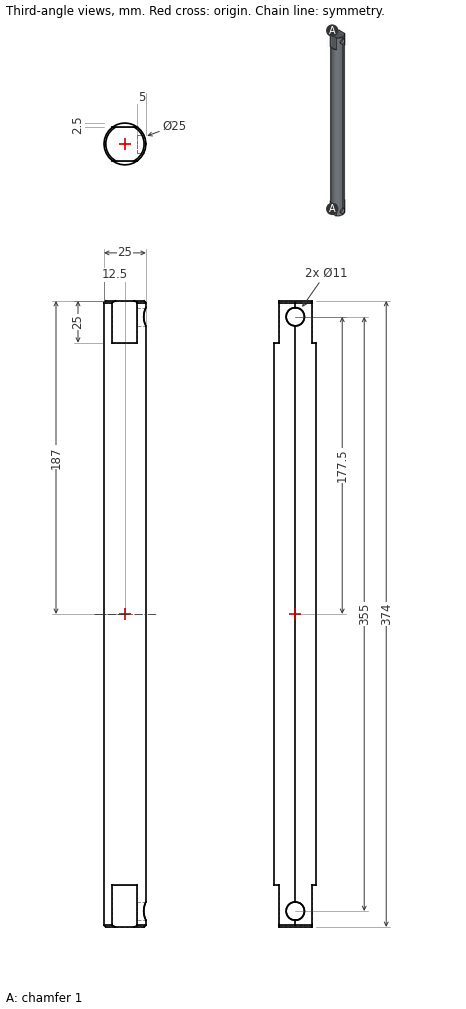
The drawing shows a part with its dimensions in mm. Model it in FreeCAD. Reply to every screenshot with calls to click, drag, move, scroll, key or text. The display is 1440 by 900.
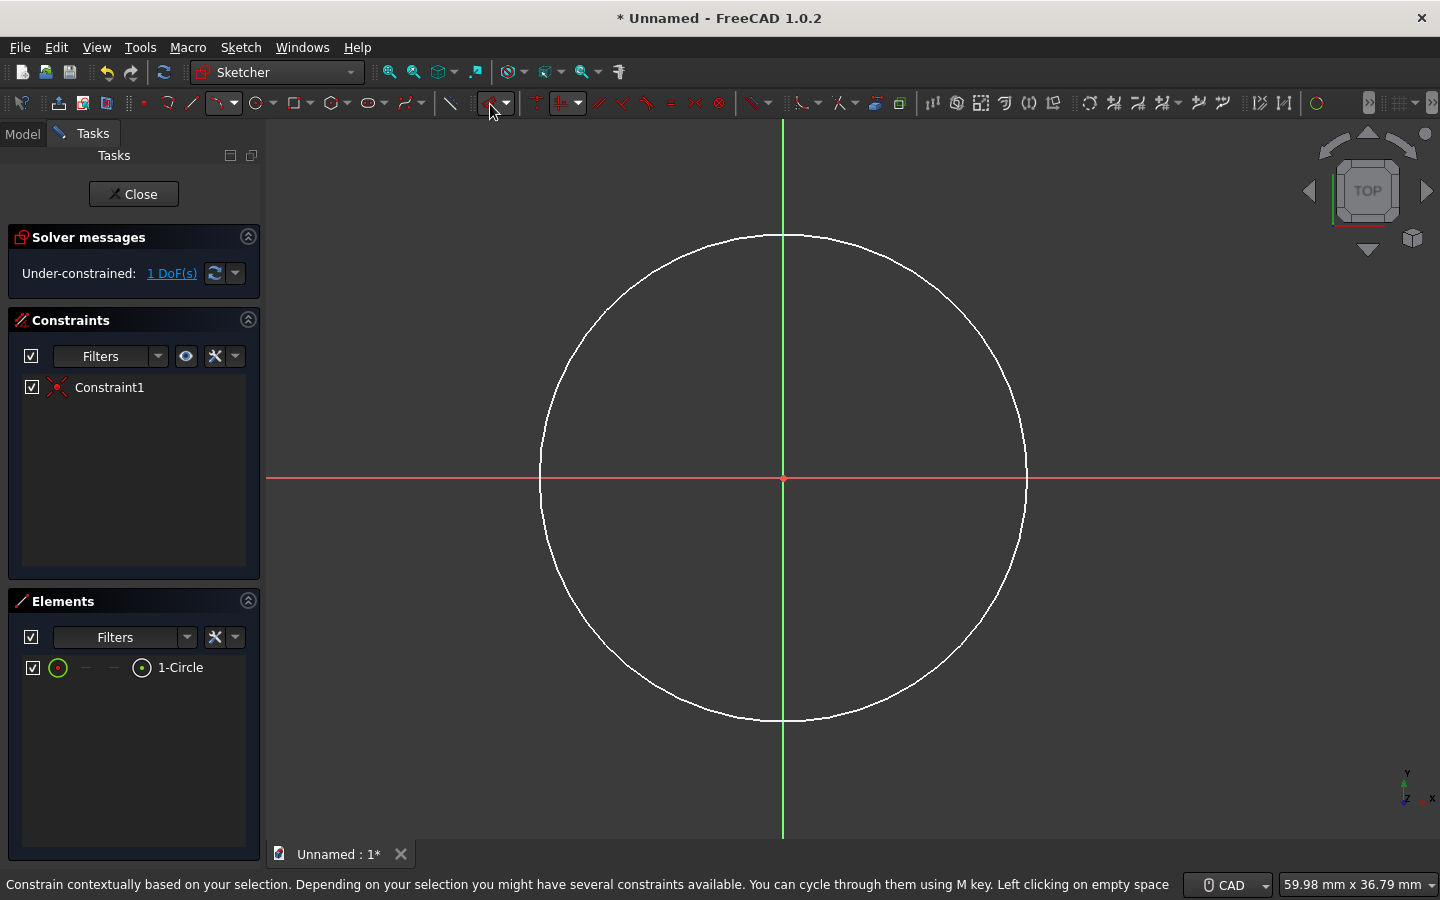
click(955, 305)
click(978, 282)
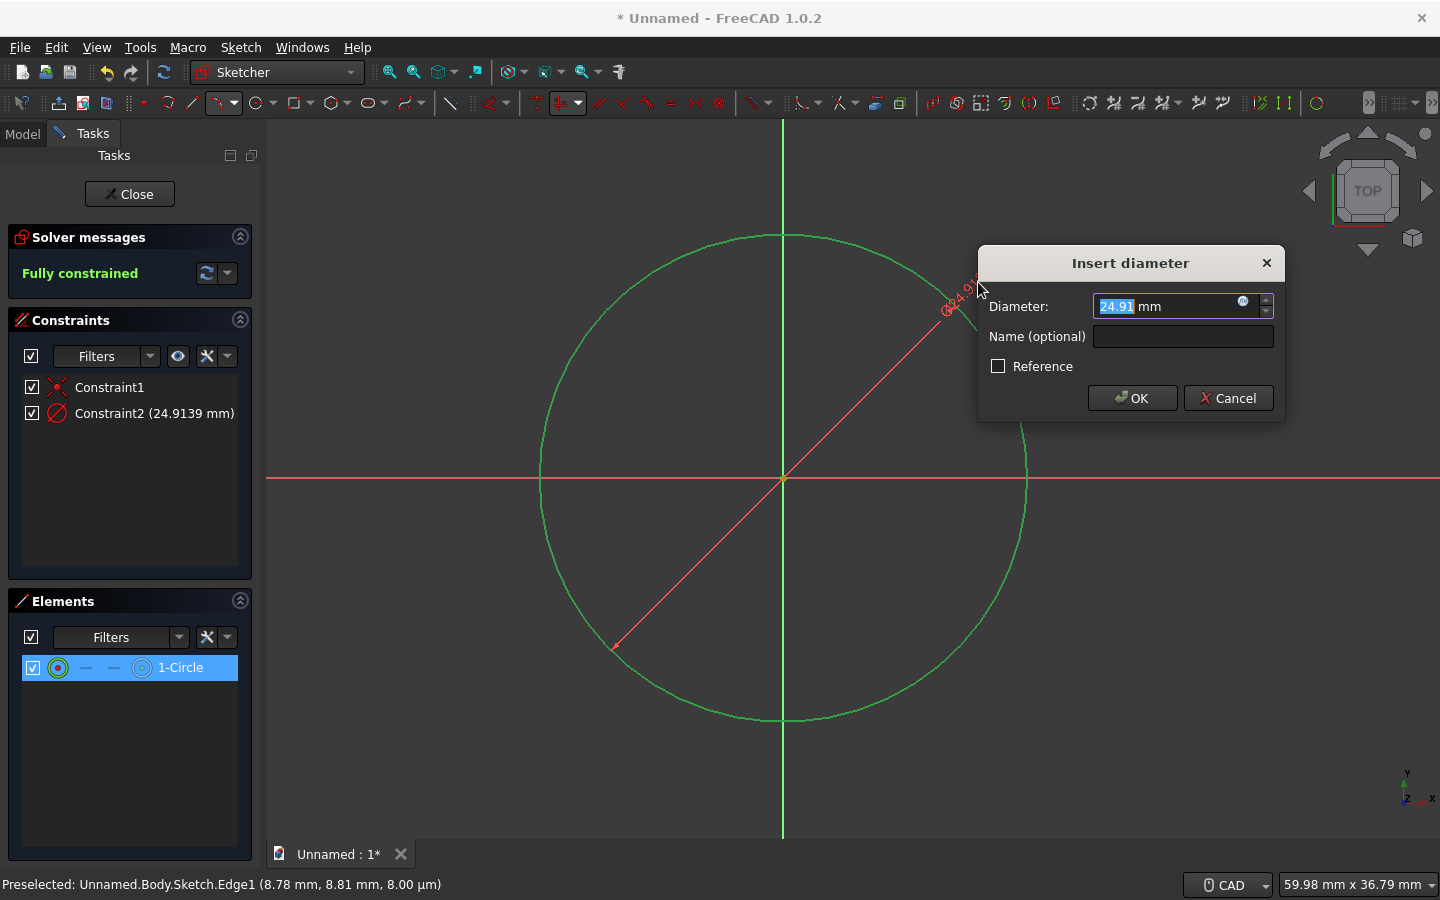
text(25)
key(Return)
key(Escape)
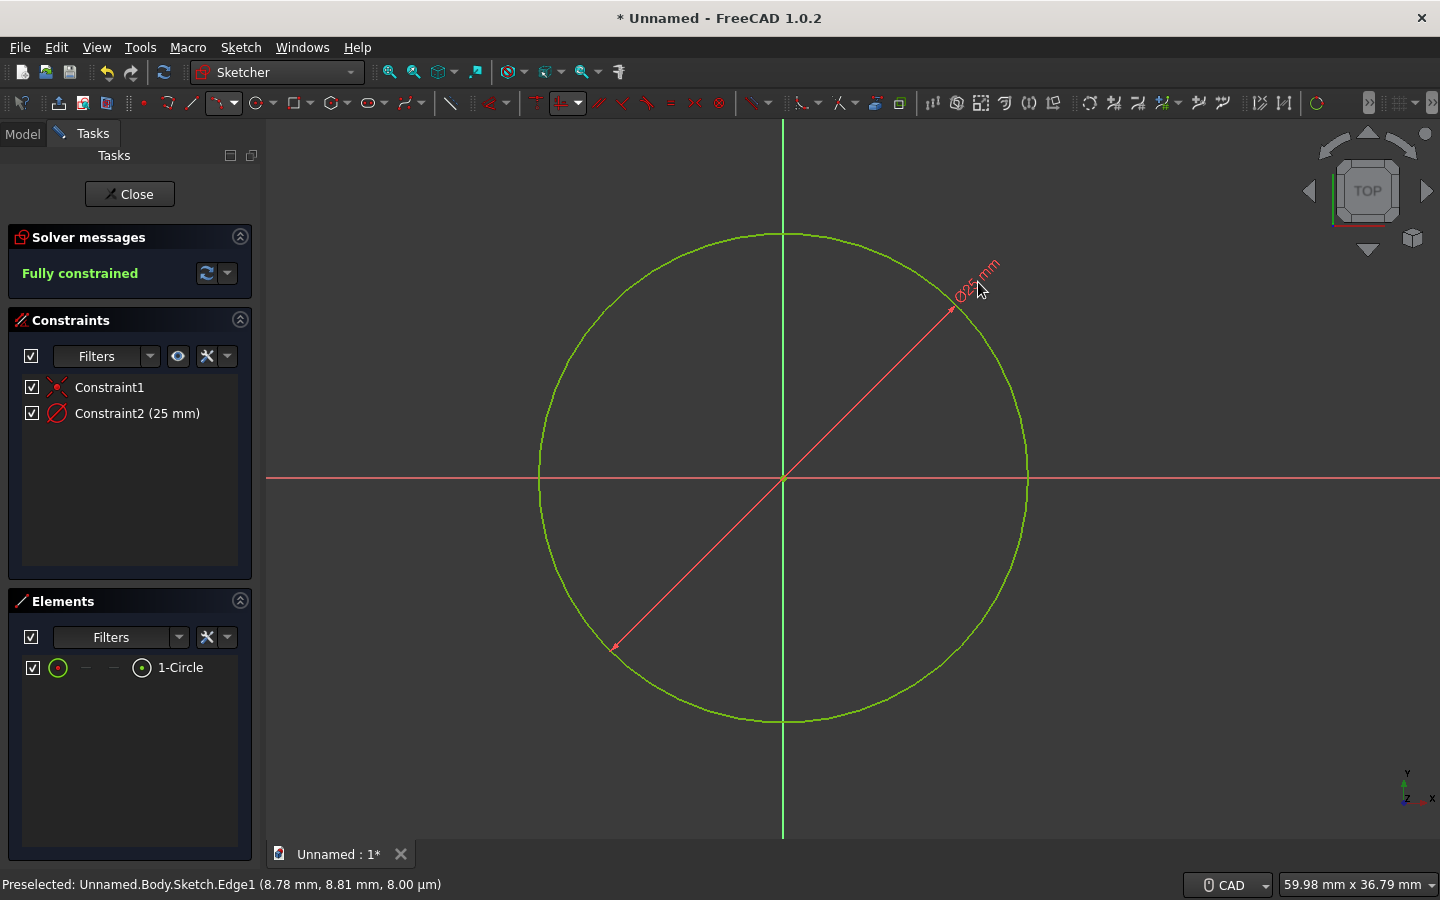
click(130, 194)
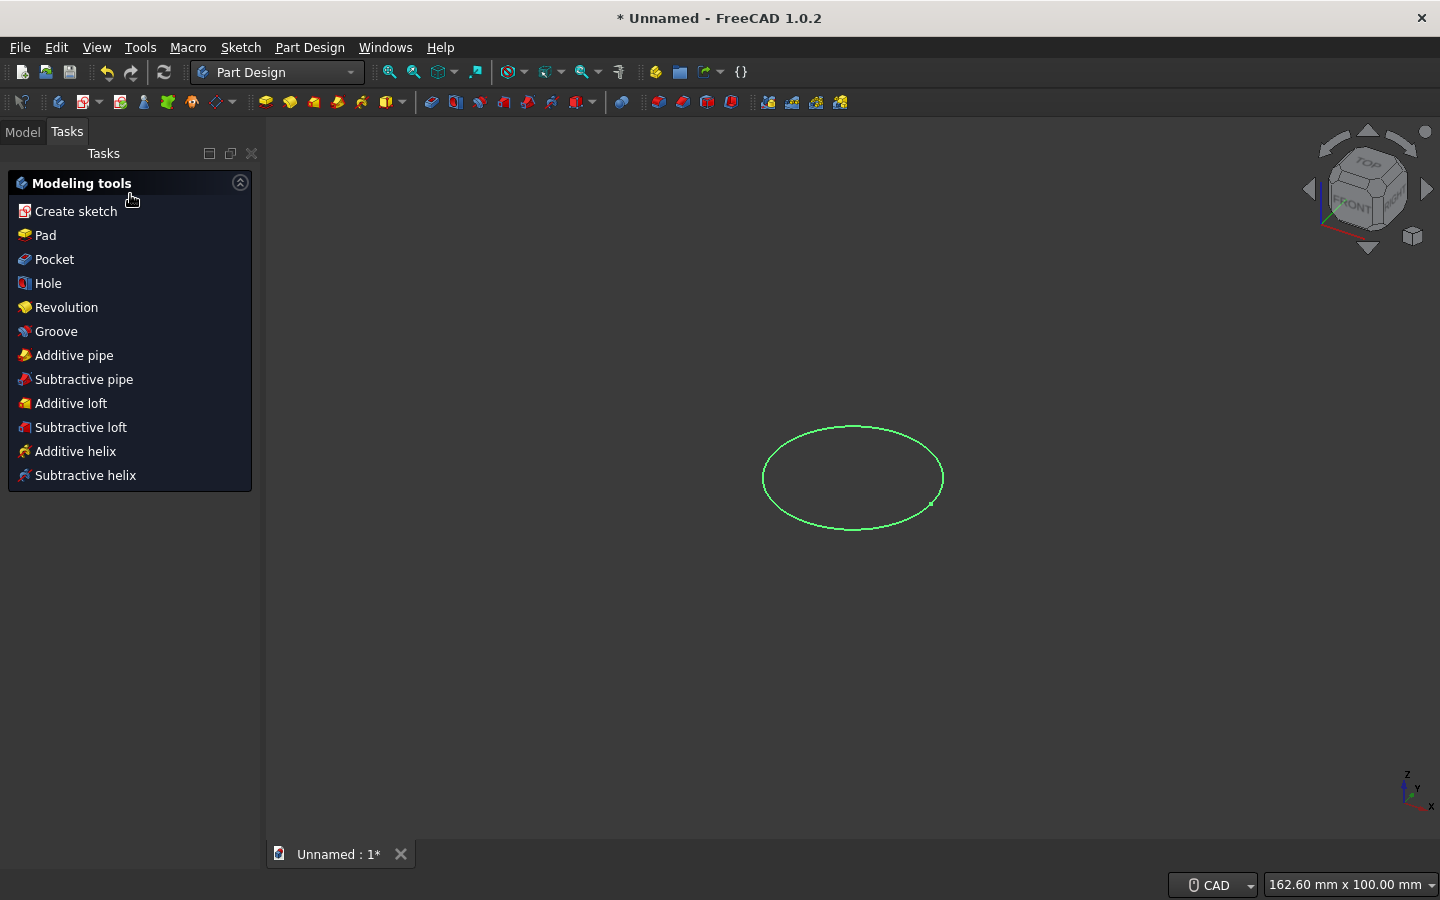
click(266, 102)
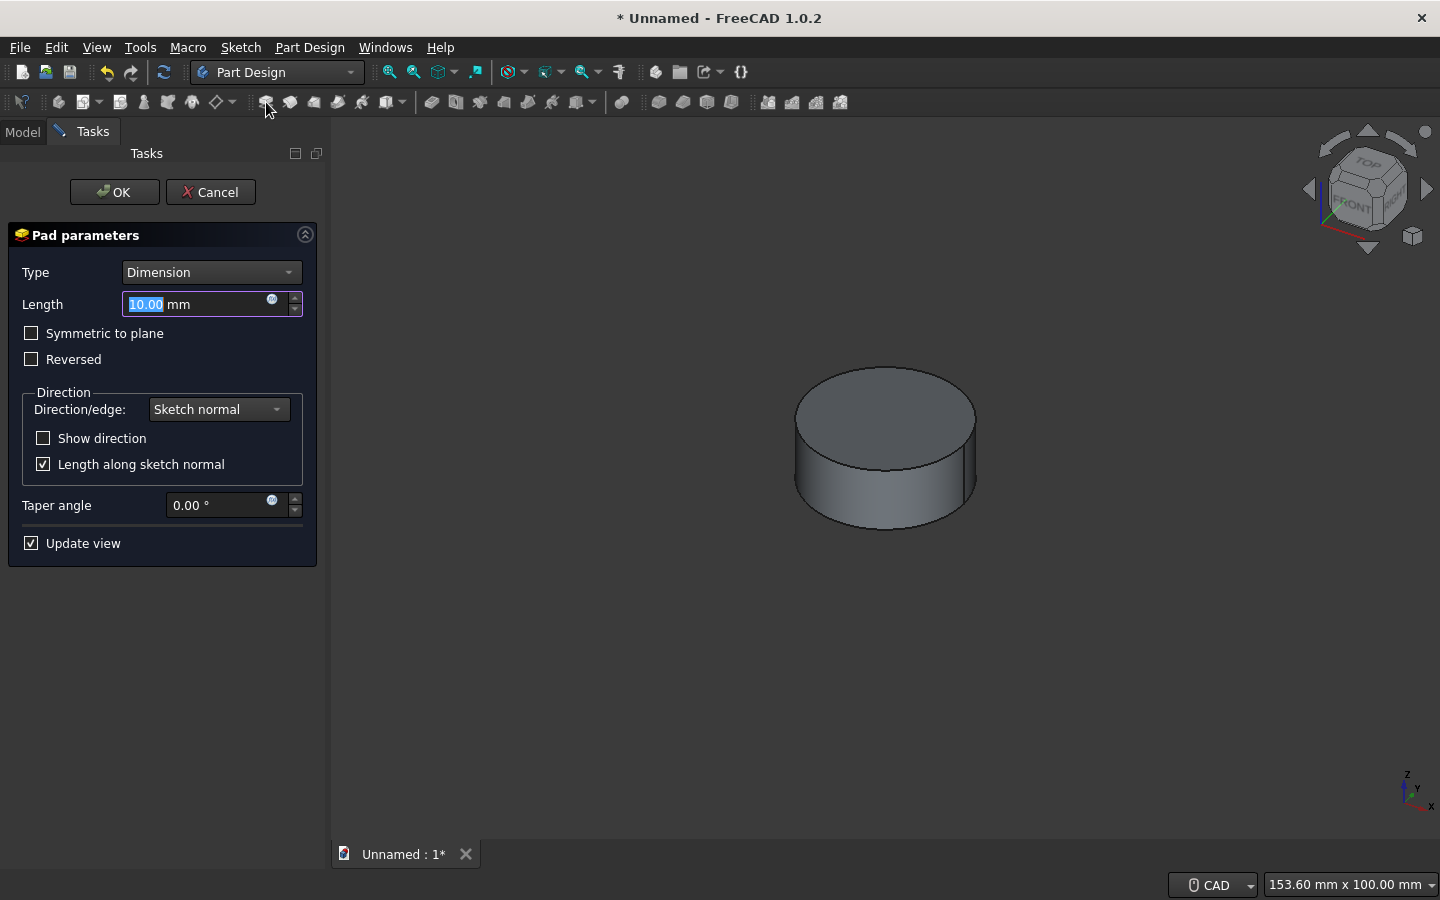
text(374)
key(Tab)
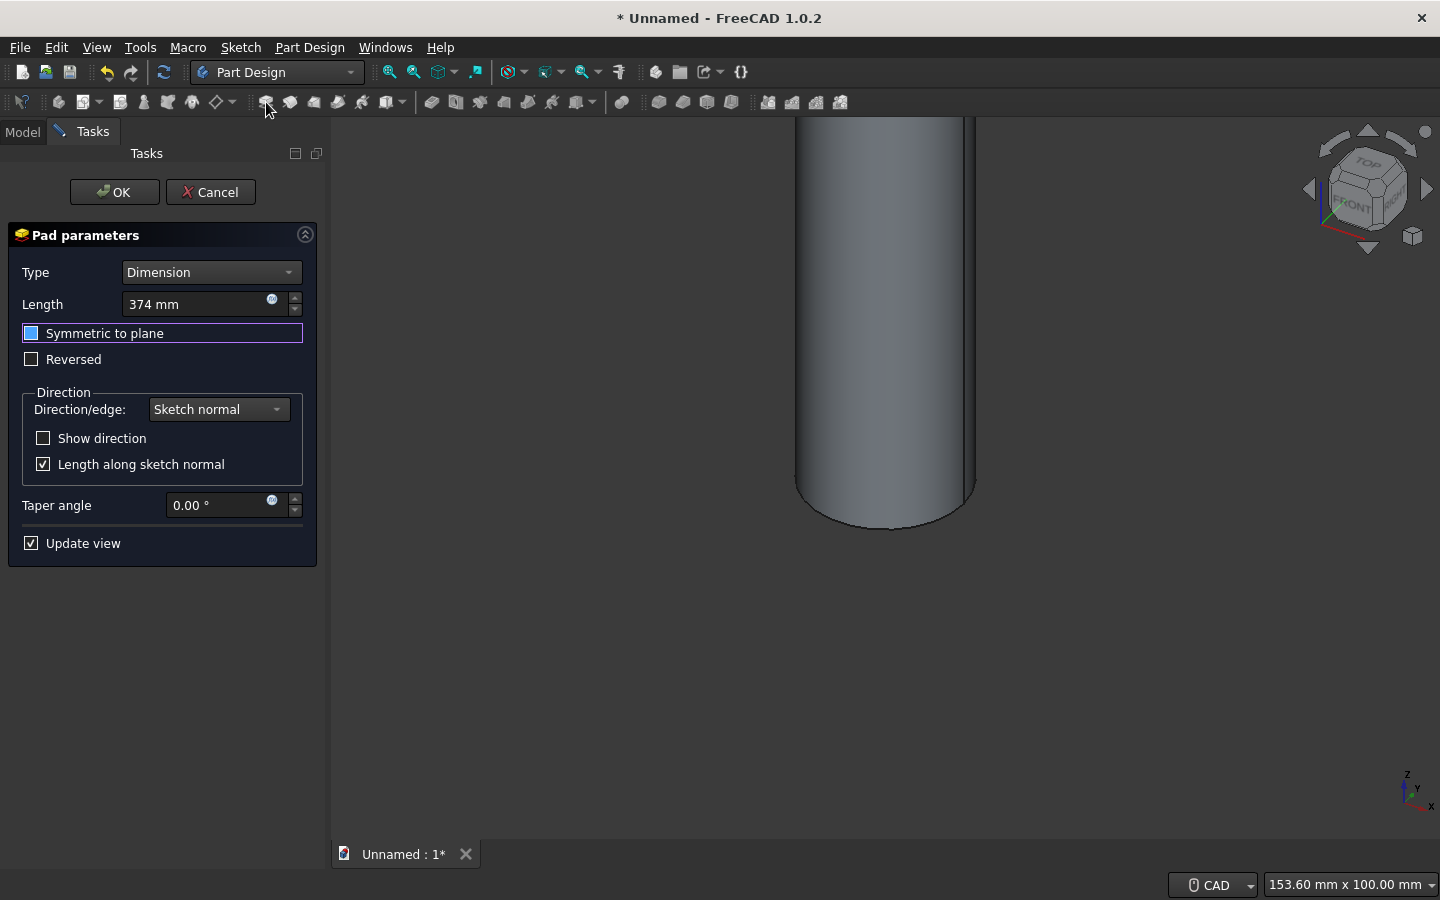
click(30, 333)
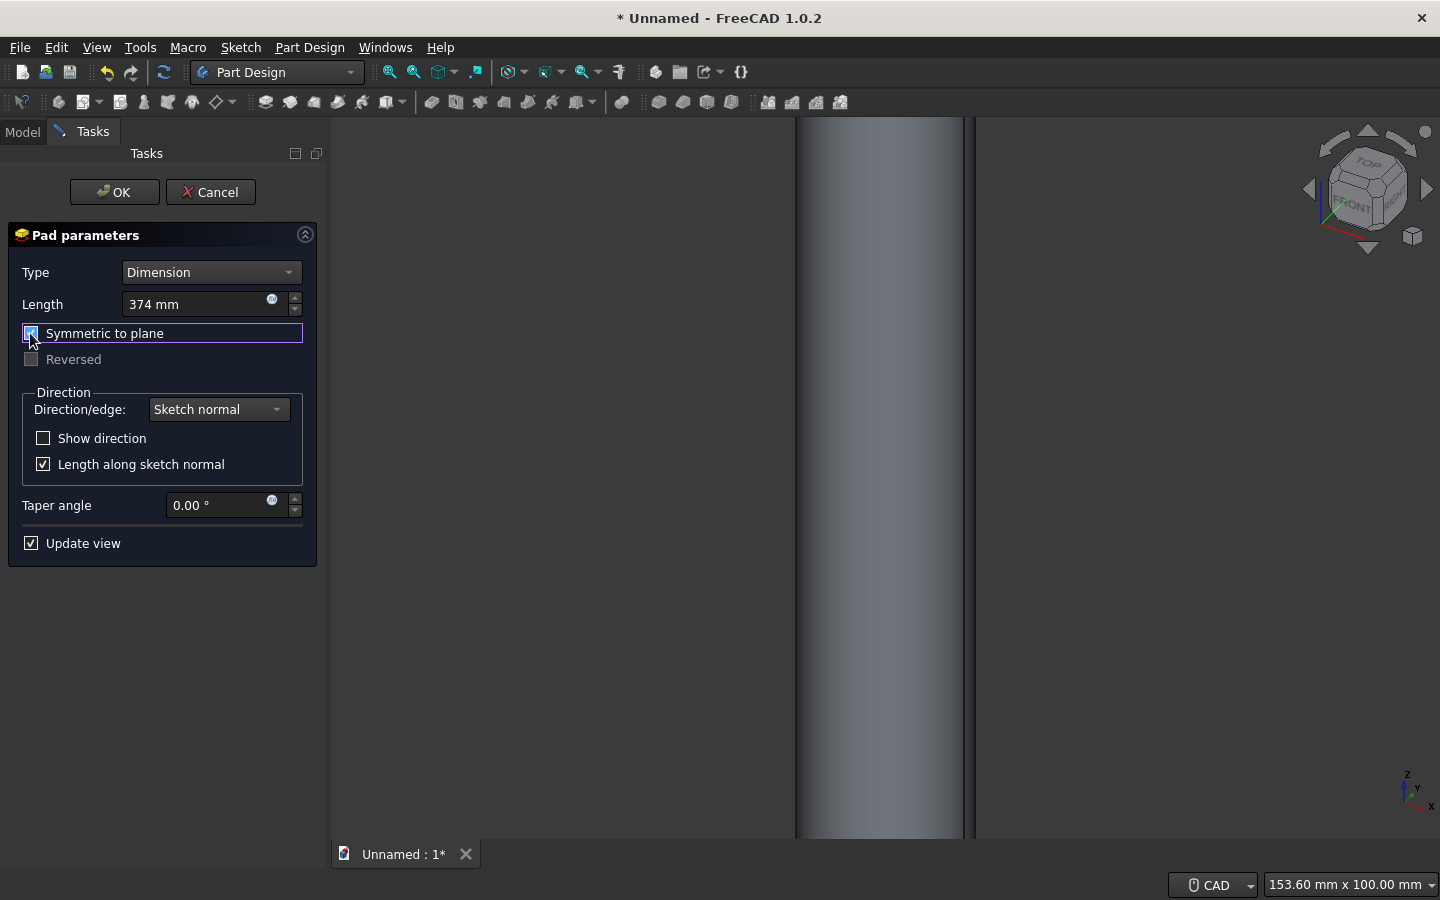
click(115, 192)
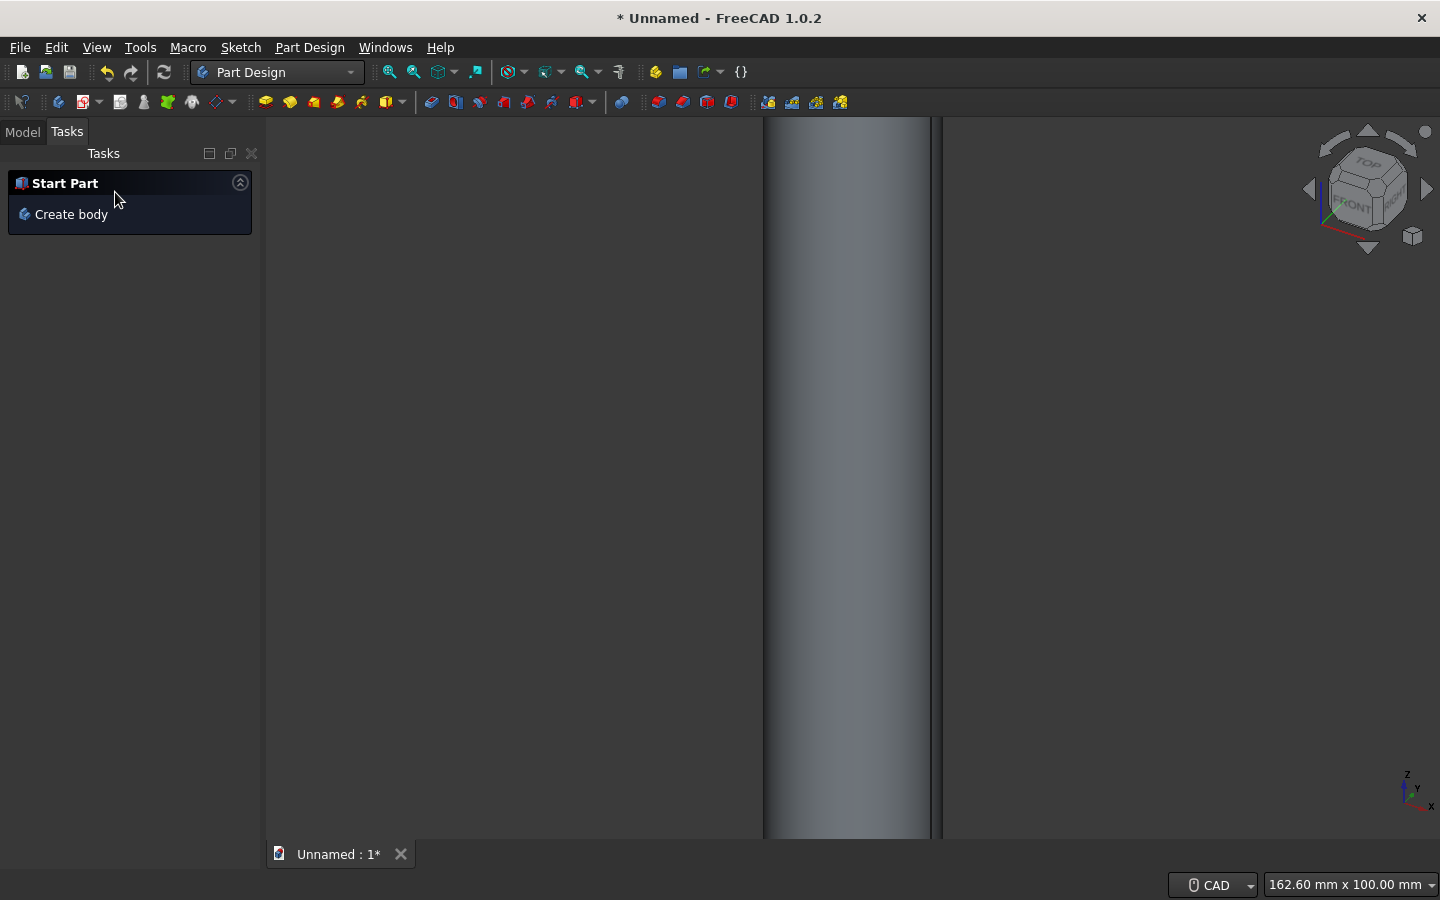
click(390, 72)